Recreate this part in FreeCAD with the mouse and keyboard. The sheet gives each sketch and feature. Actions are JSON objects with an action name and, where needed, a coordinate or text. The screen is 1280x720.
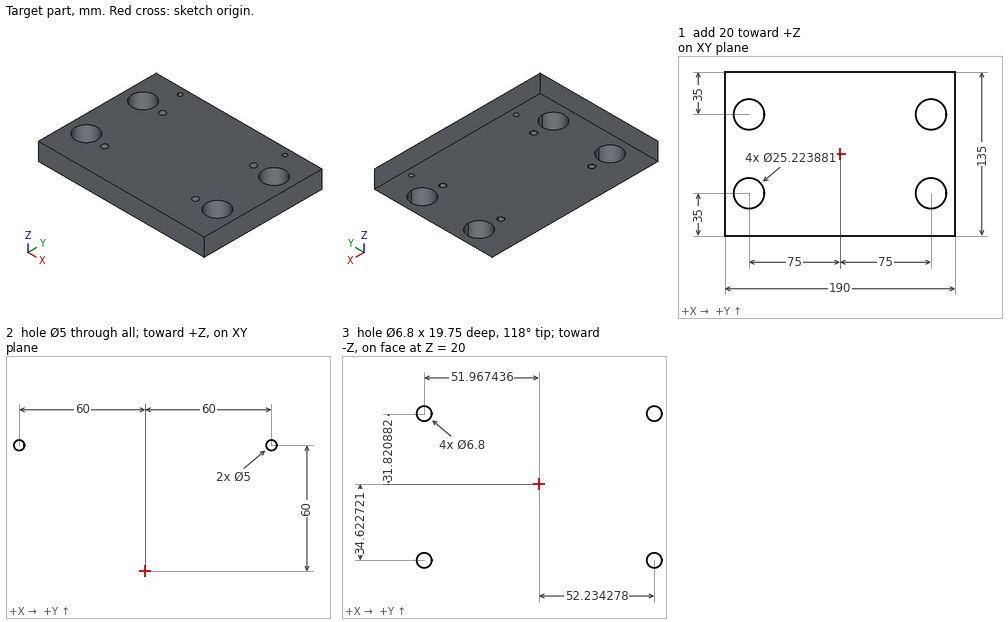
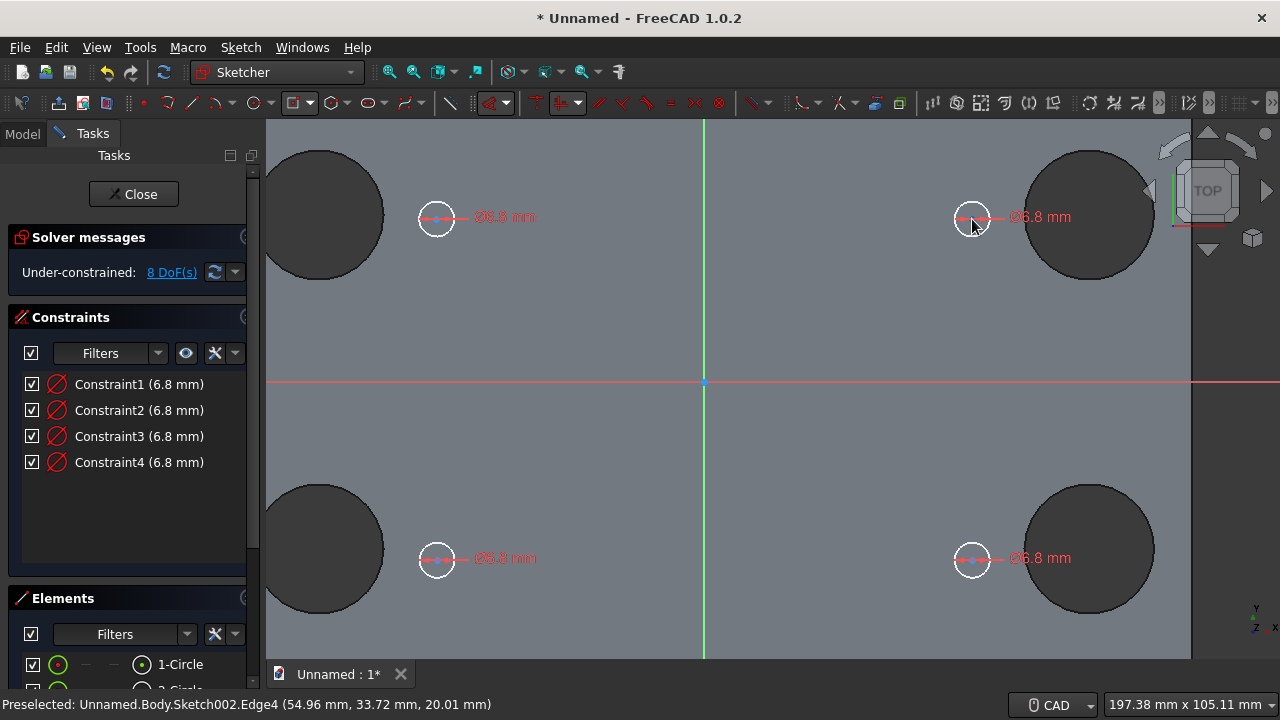
{"action": "left_click", "coordinate": [437, 219]}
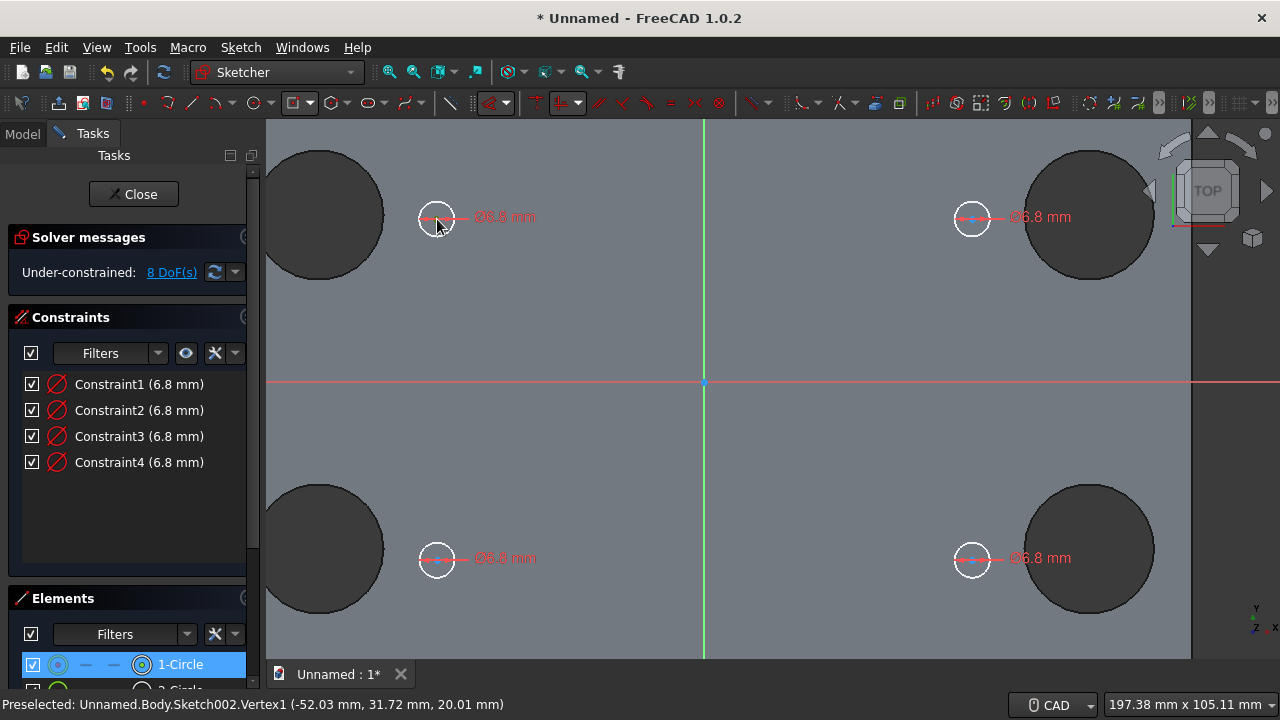
{"action": "left_click", "coordinate": [437, 560]}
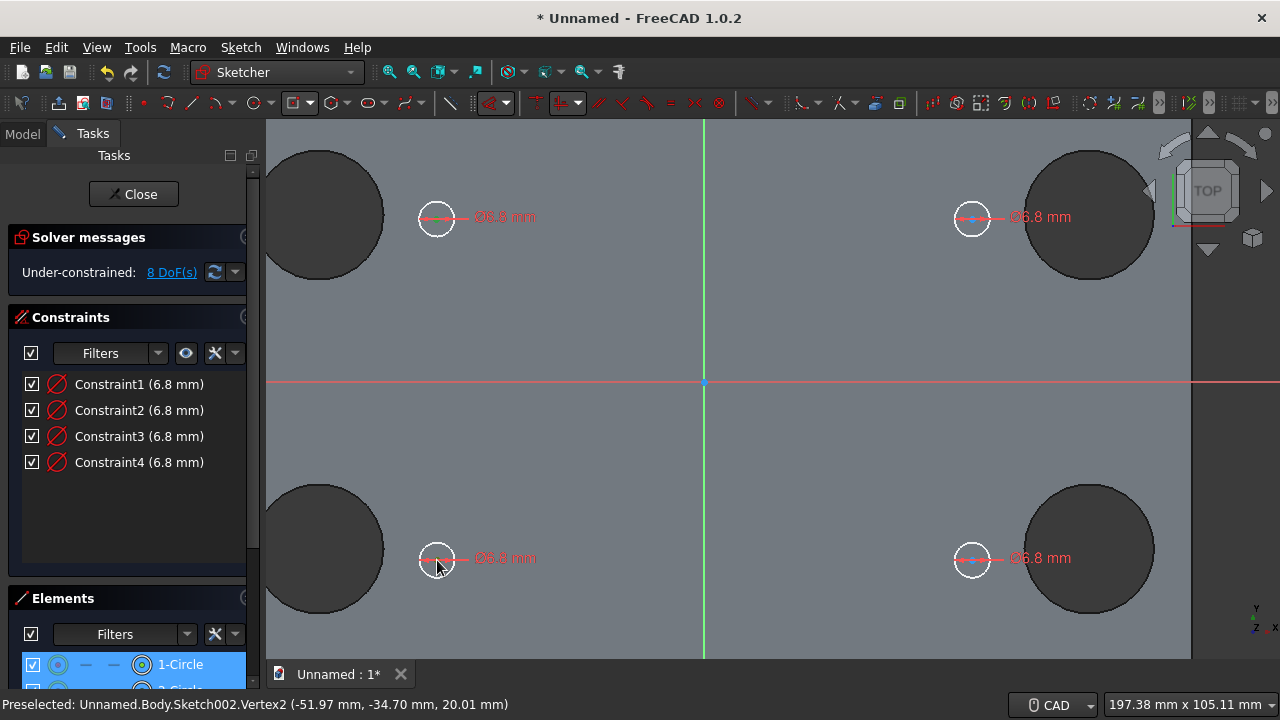
{"action": "left_click", "coordinate": [580, 104]}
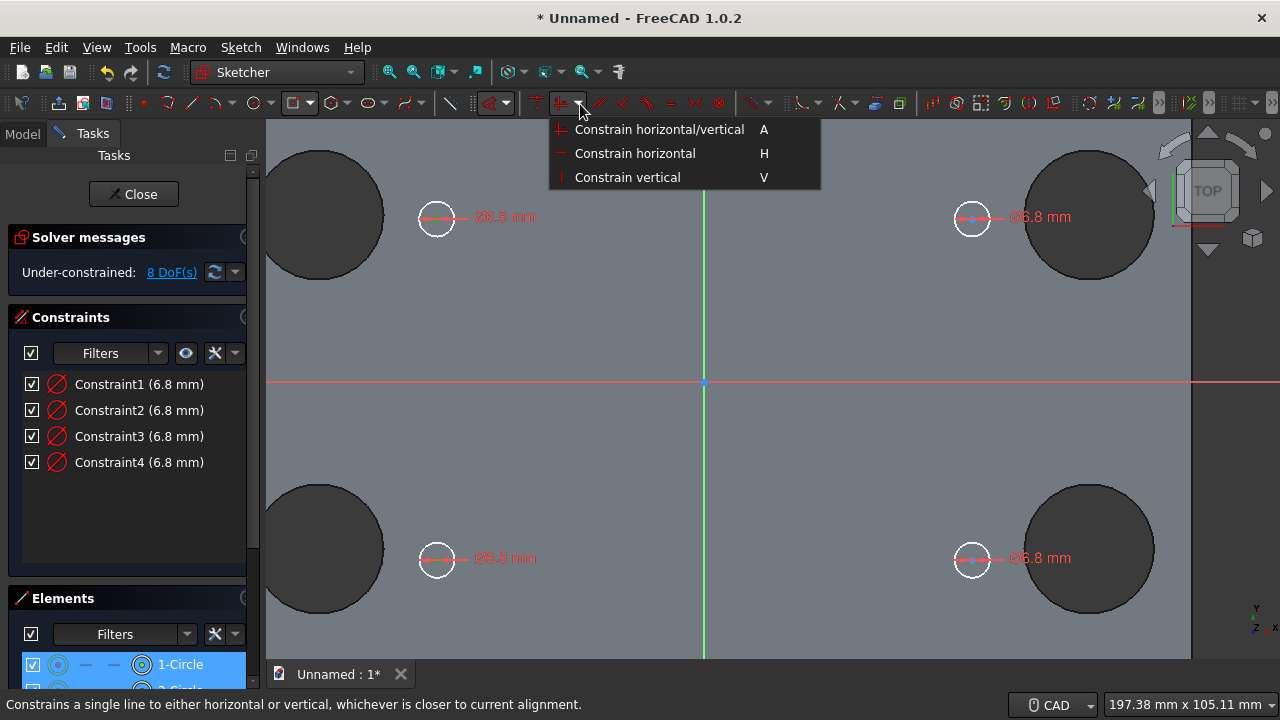
{"action": "left_click", "coordinate": [685, 177]}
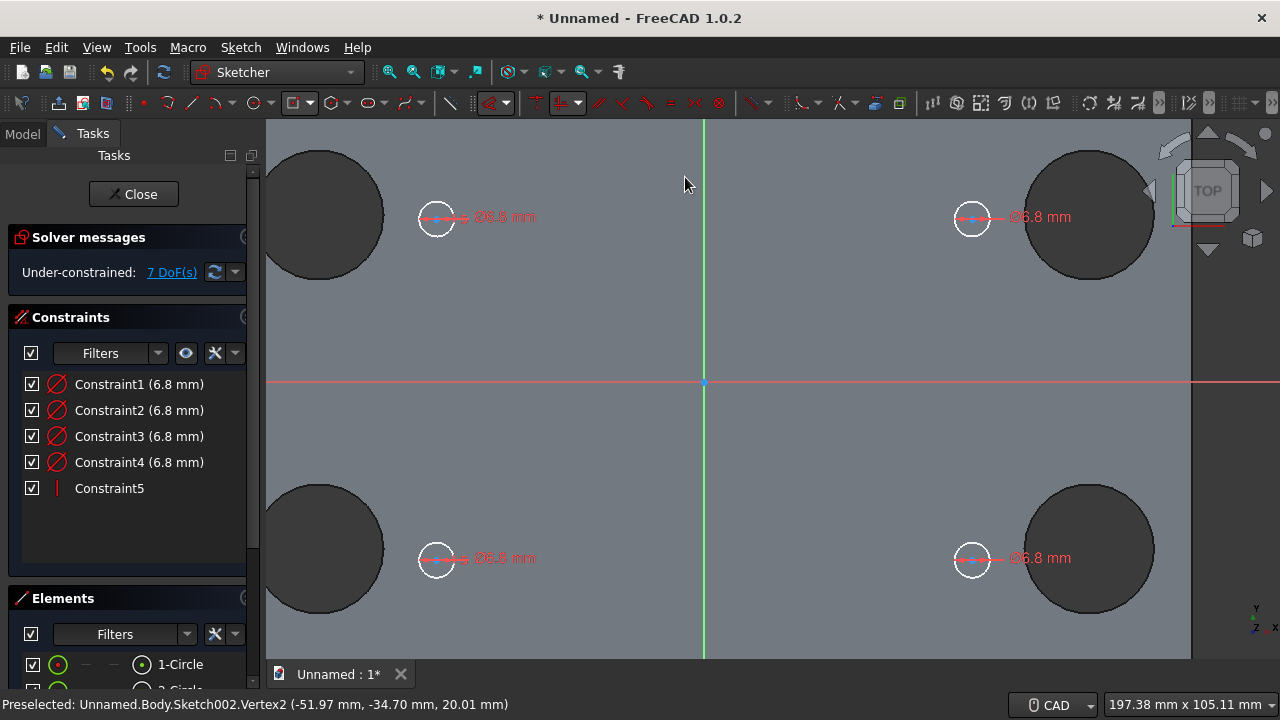
{"action": "left_click", "coordinate": [437, 560]}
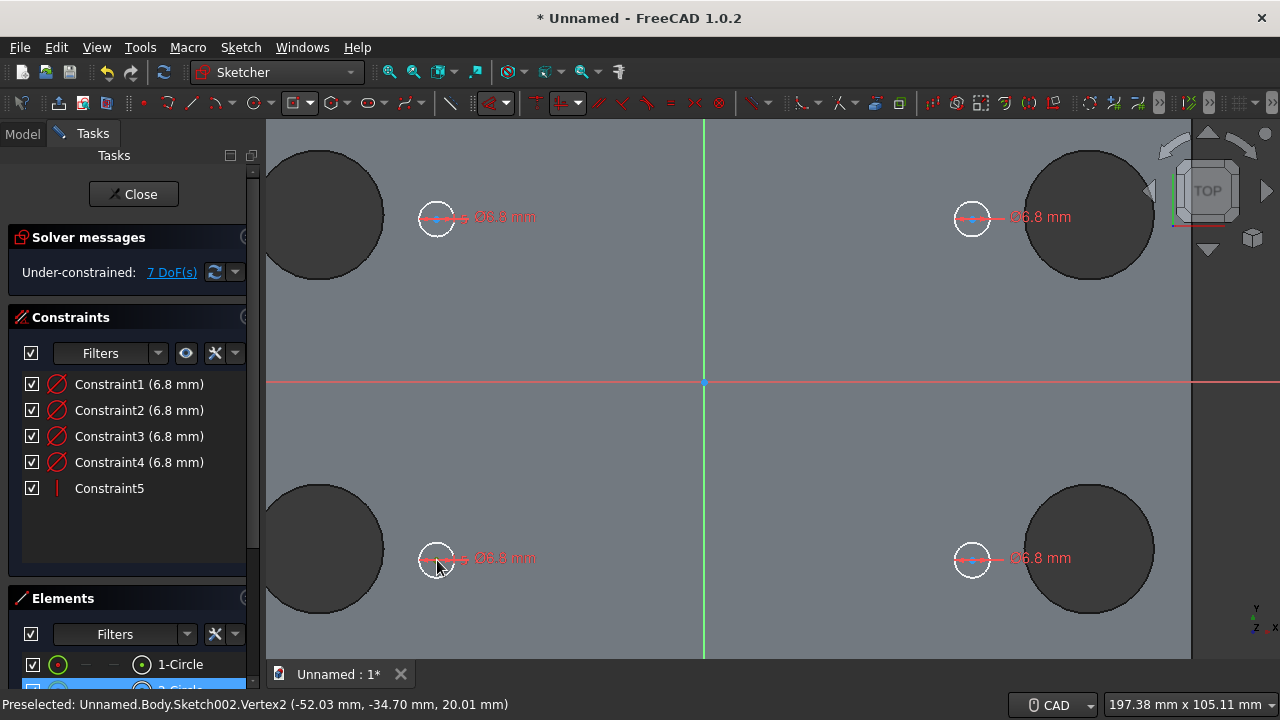
{"action": "left_click", "coordinate": [972, 560]}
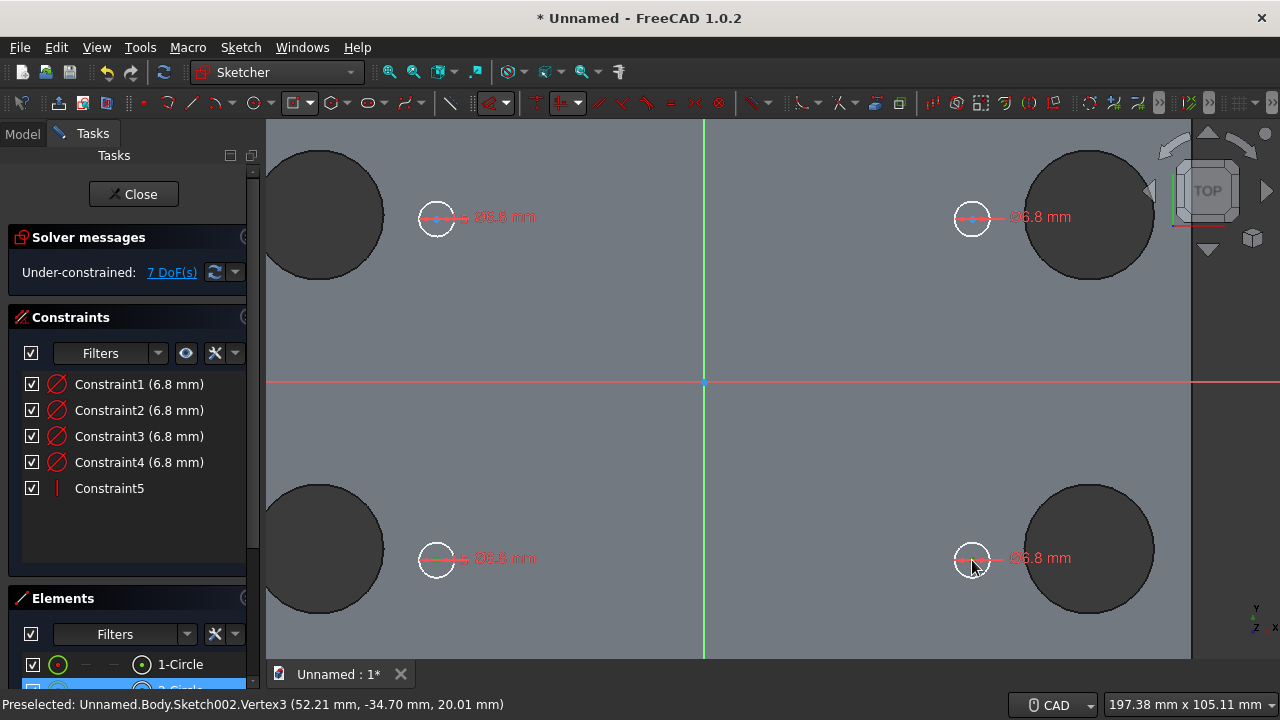
{"action": "key", "text": "h"}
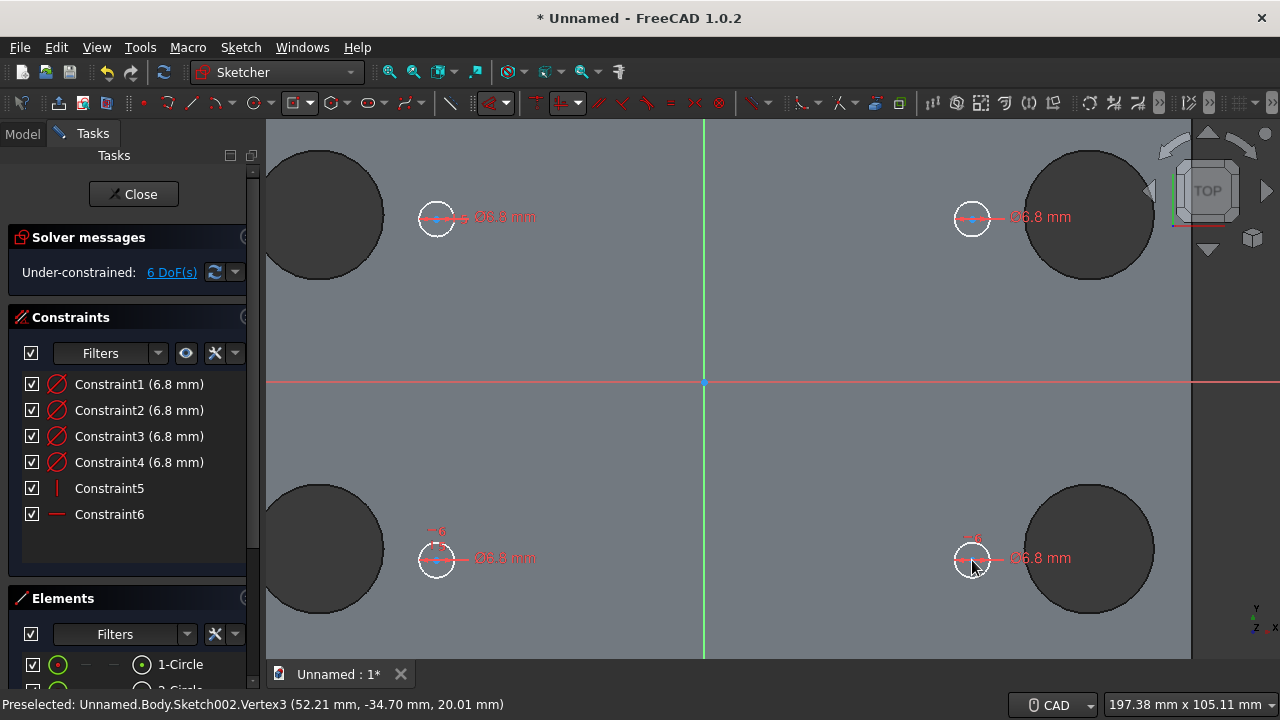
{"action": "left_click", "coordinate": [972, 560]}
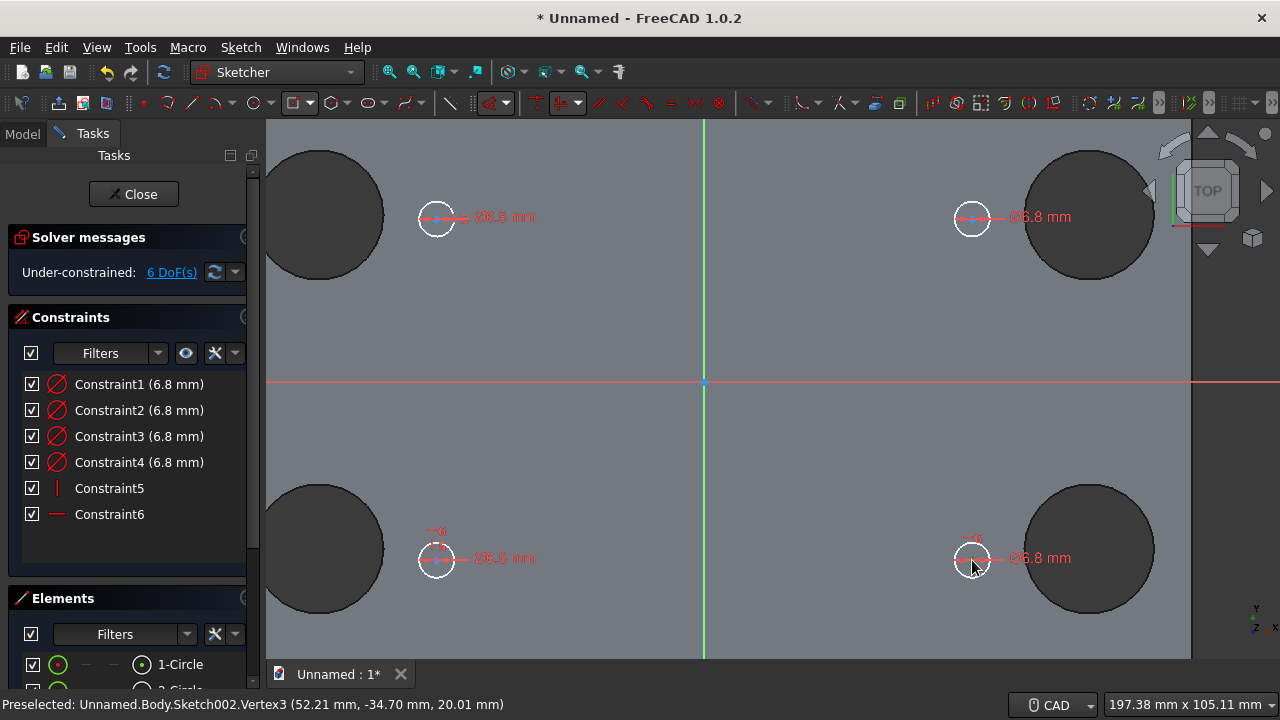
{"action": "left_click", "coordinate": [972, 219]}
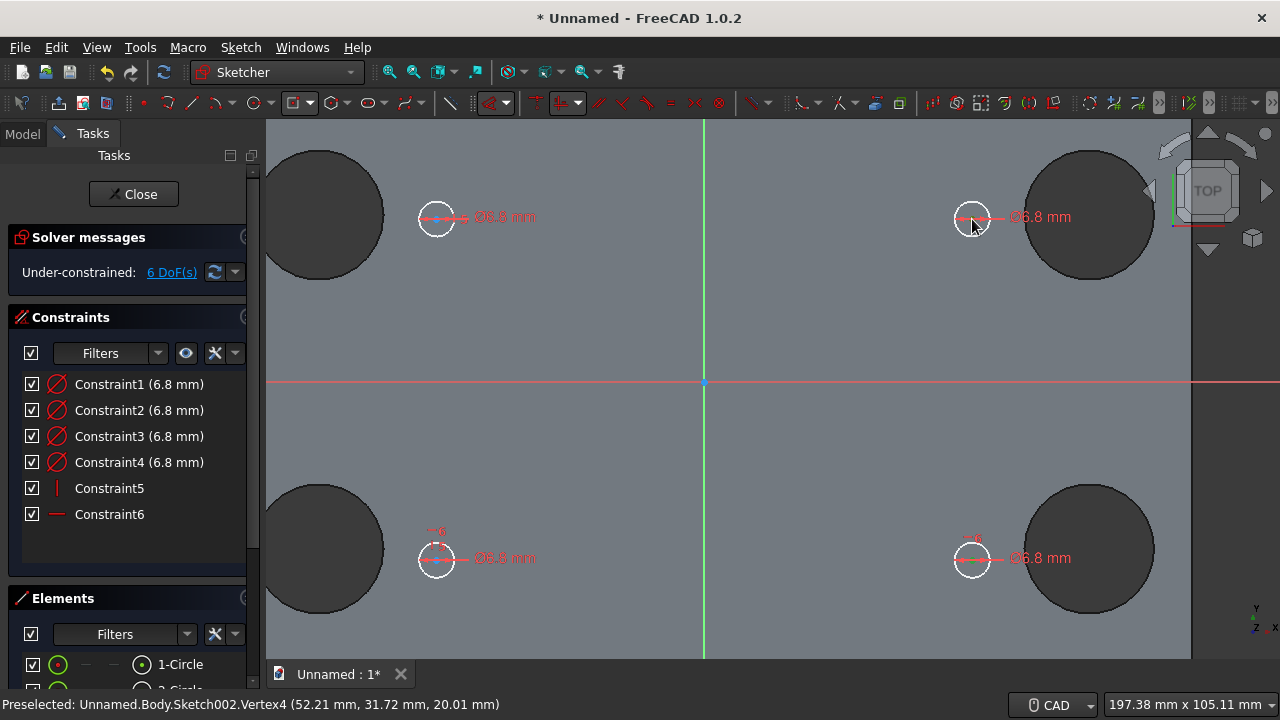
{"action": "key", "text": "v"}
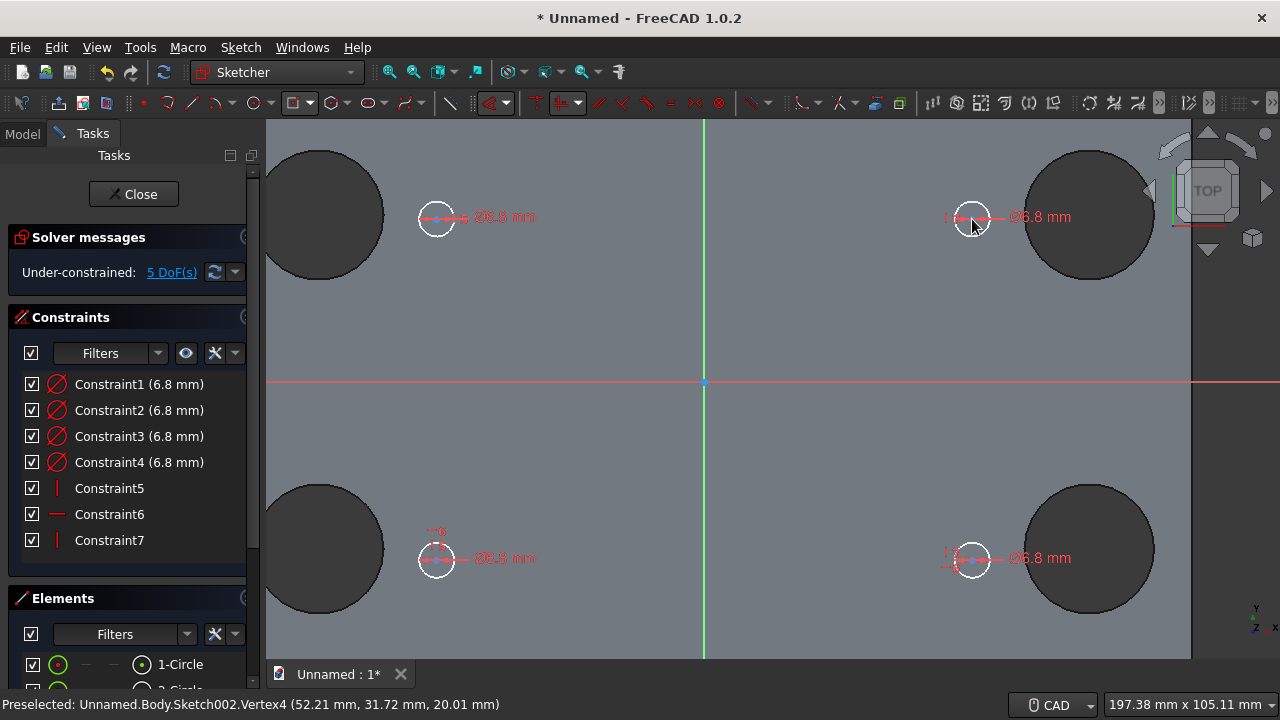
{"action": "left_click", "coordinate": [437, 219]}